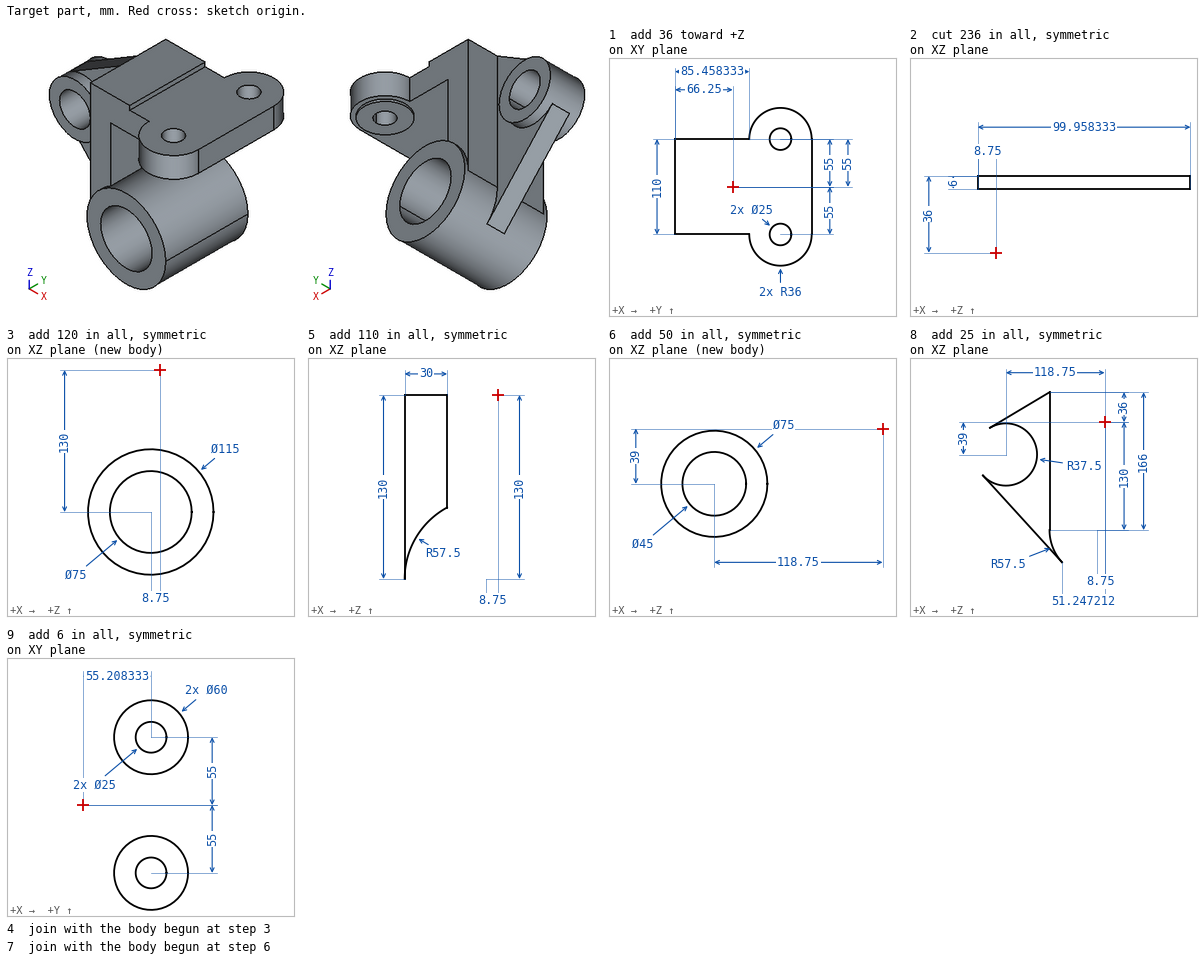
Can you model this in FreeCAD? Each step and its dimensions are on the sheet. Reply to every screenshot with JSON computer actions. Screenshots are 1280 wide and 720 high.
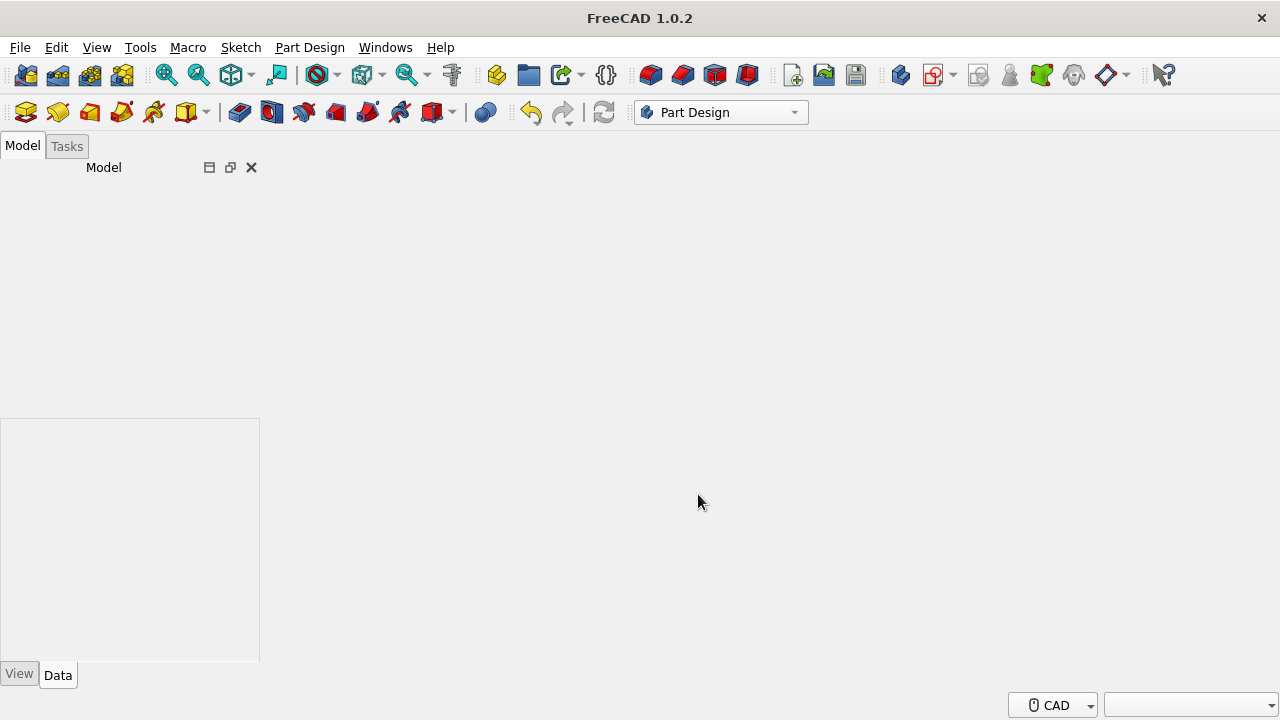
{"action": "left_click", "coordinate": [792, 76]}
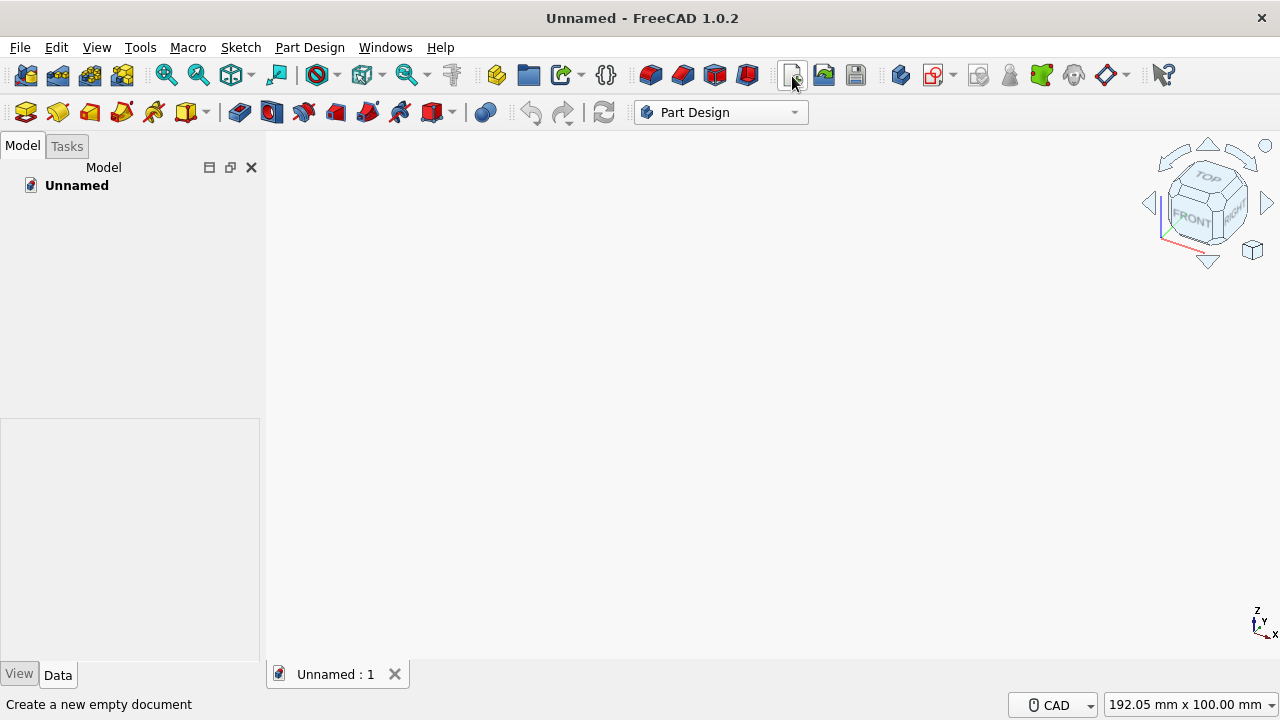
{"action": "left_click", "coordinate": [934, 76]}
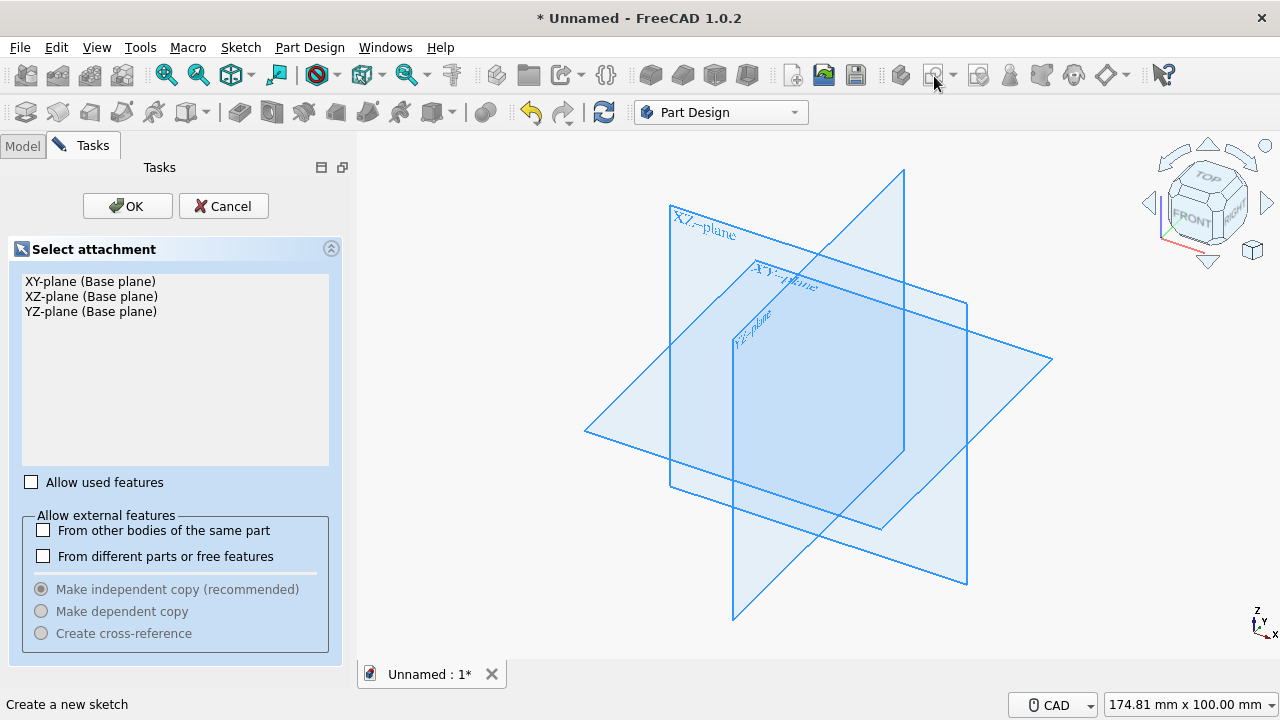
{"action": "left_click", "coordinate": [82, 282]}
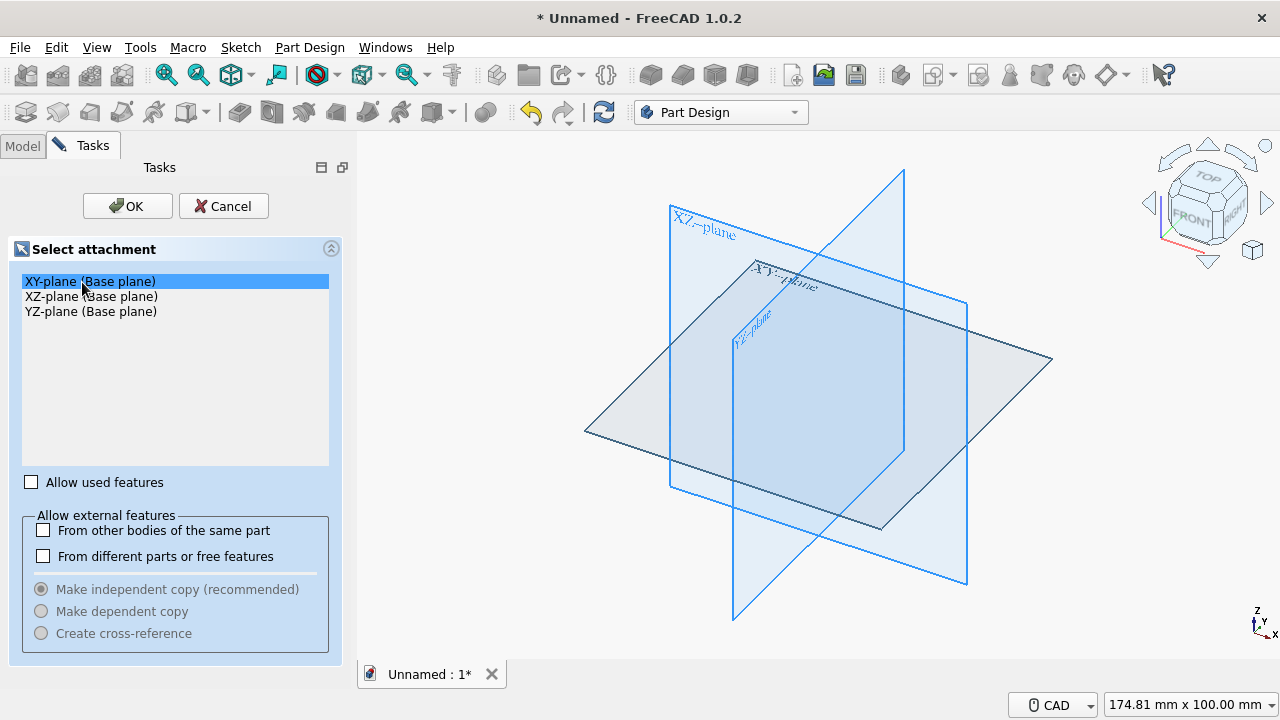
{"action": "left_click", "coordinate": [128, 206]}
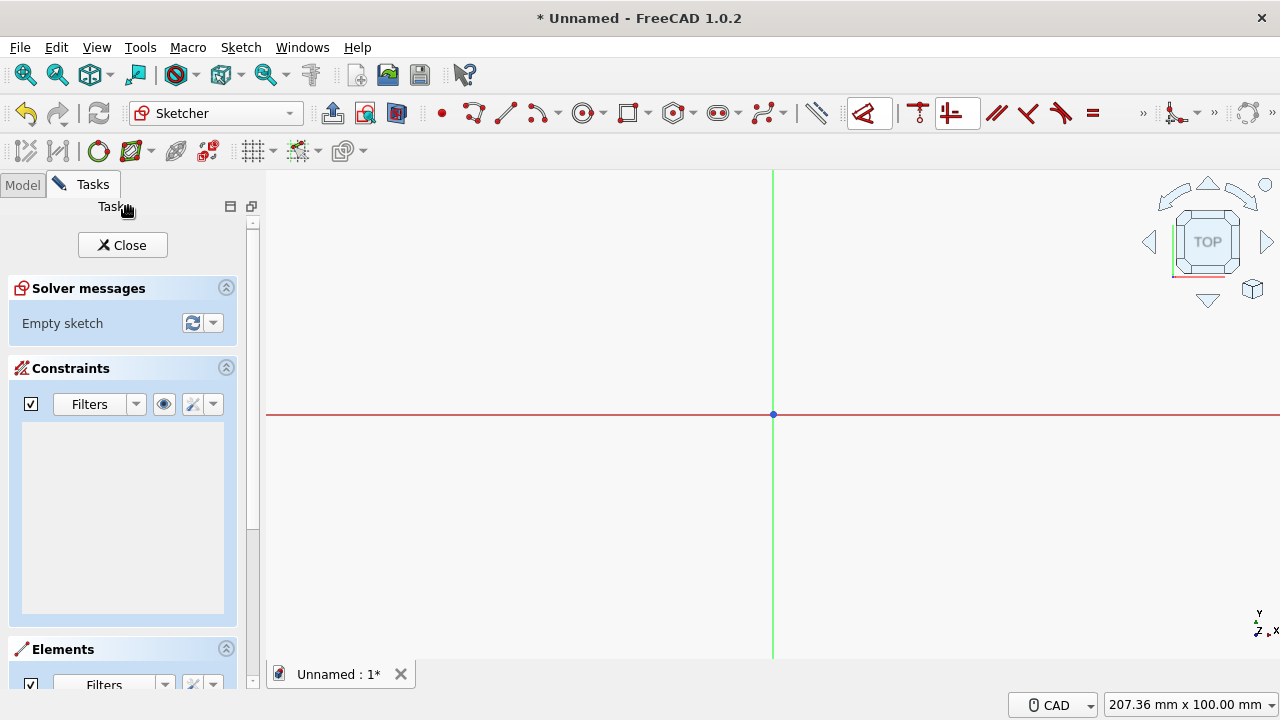
{"action": "scroll", "coordinate": [629, 414], "scroll_direction": "down", "scroll_amount": 5}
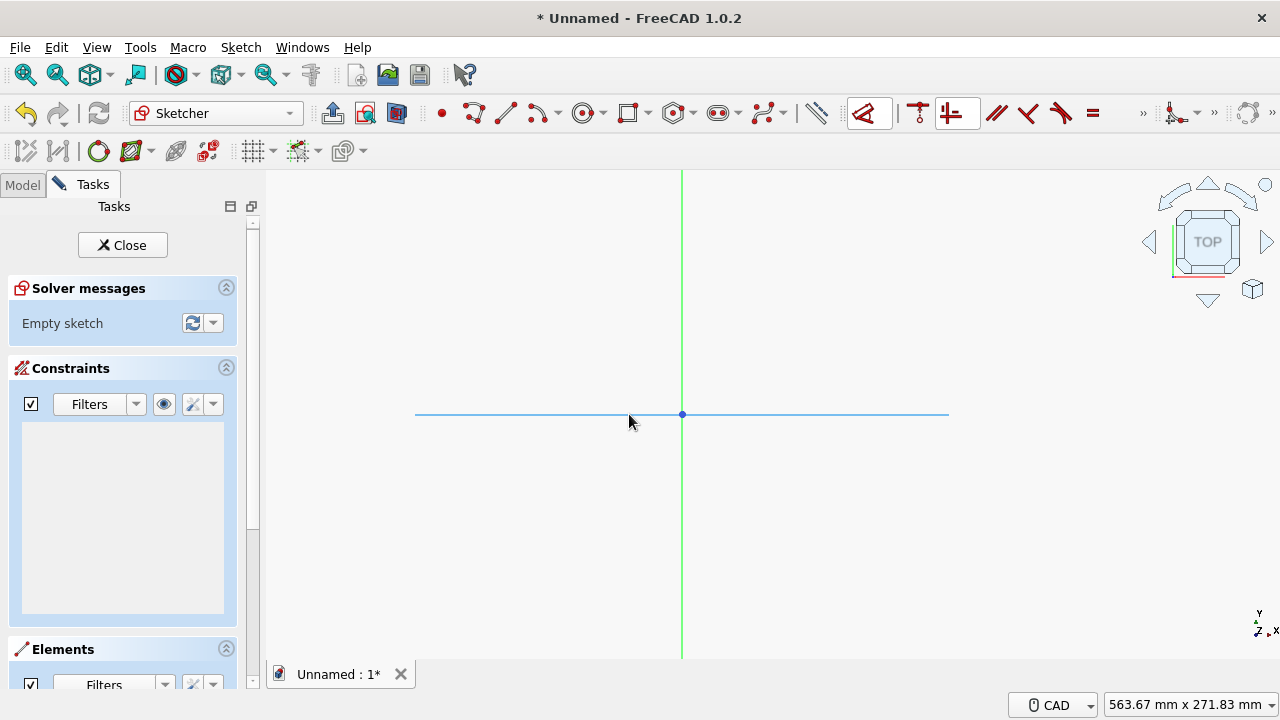
{"action": "left_click", "coordinate": [474, 114]}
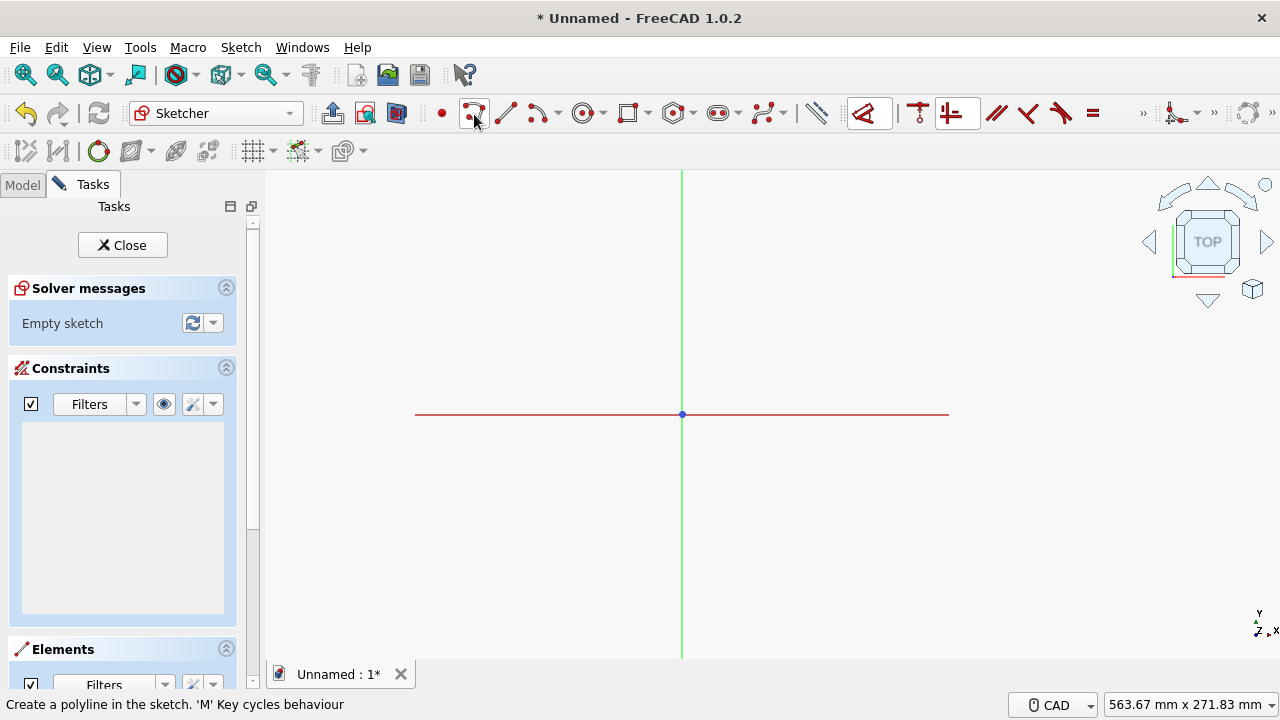
{"action": "left_click", "coordinate": [717, 316]}
{"action": "left_click", "coordinate": [563, 316]}
{"action": "left_click", "coordinate": [563, 513]}
{"action": "left_click", "coordinate": [717, 513]}
{"action": "right_click", "coordinate": [717, 513]}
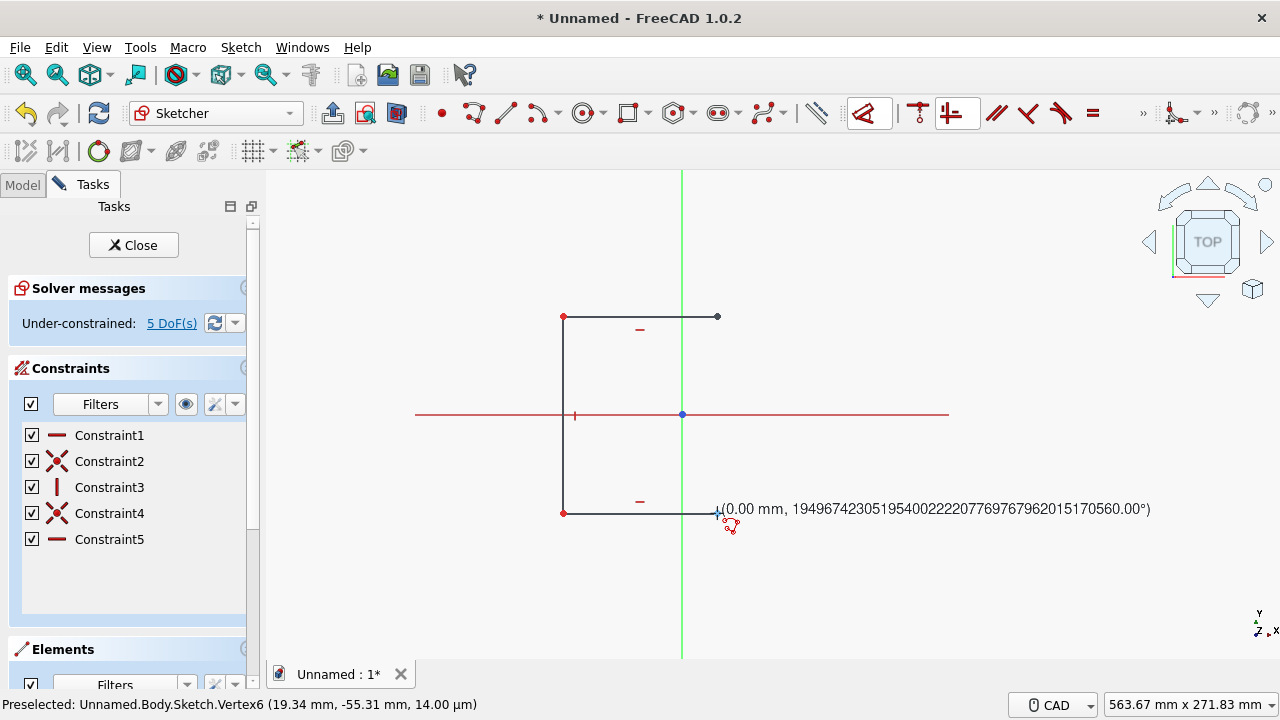
{"action": "left_click", "coordinate": [506, 114]}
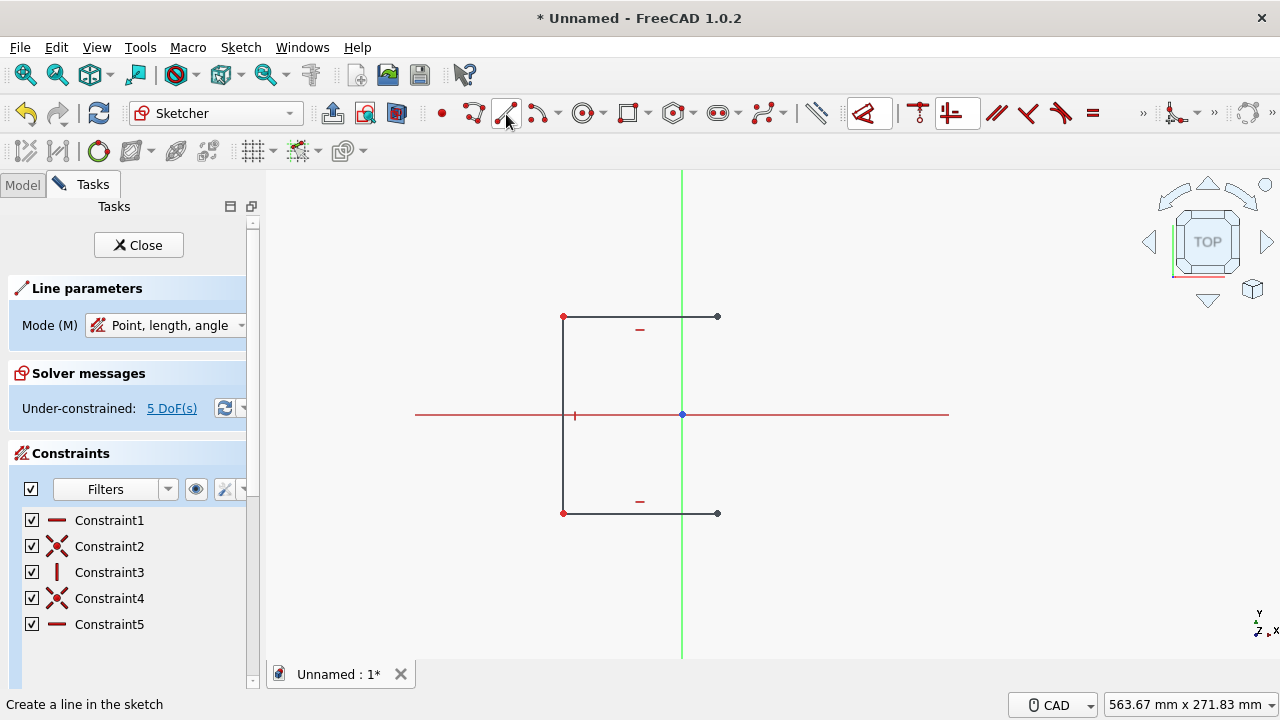
{"action": "left_click", "coordinate": [846, 513]}
{"action": "left_click", "coordinate": [846, 316]}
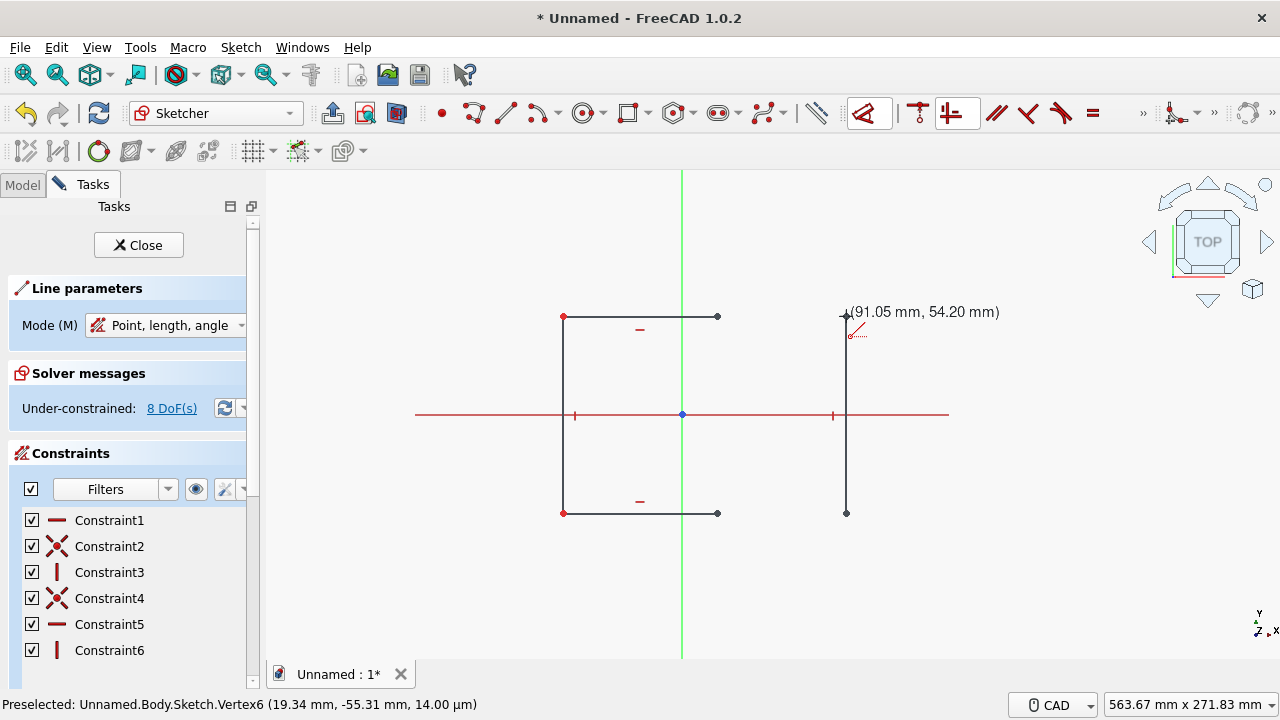
{"action": "left_click", "coordinate": [560, 114]}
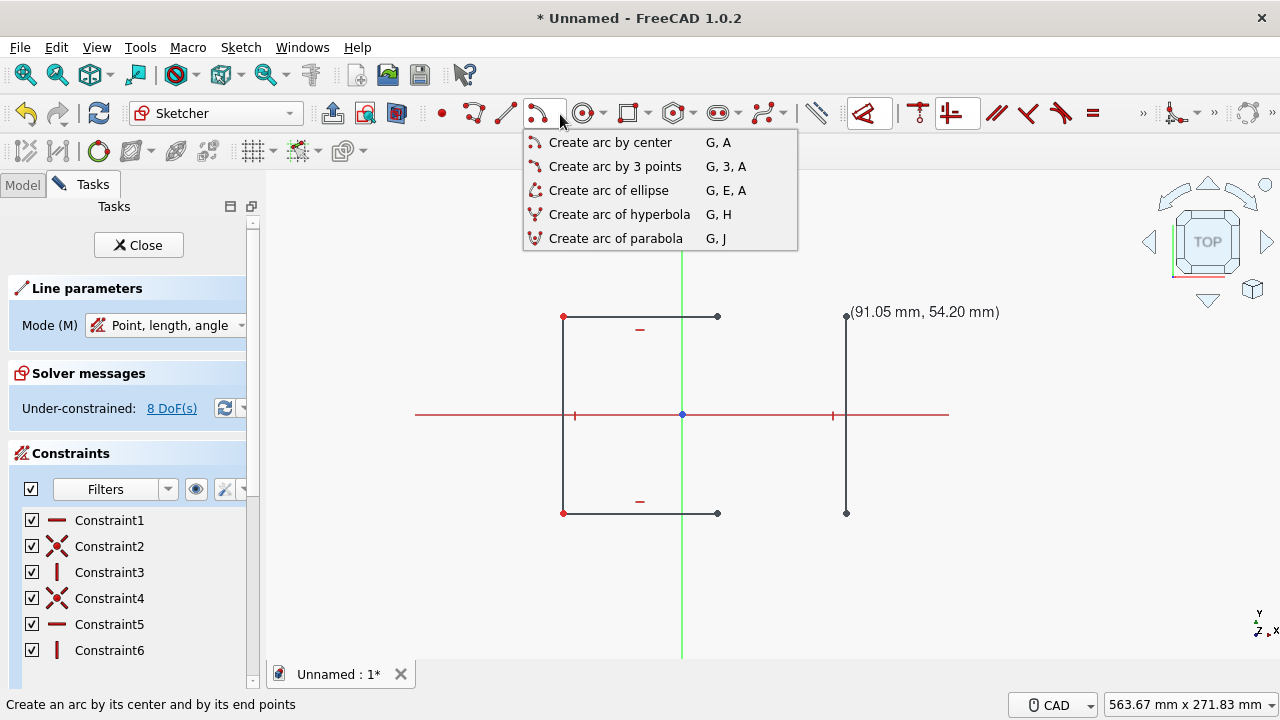
{"action": "left_click", "coordinate": [660, 166]}